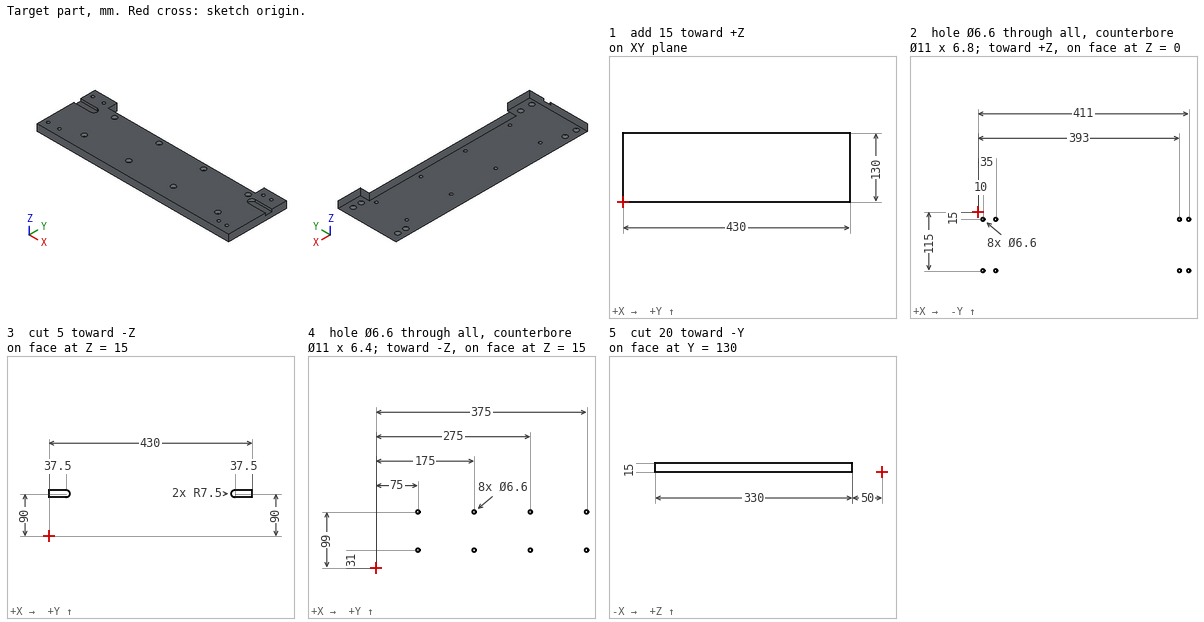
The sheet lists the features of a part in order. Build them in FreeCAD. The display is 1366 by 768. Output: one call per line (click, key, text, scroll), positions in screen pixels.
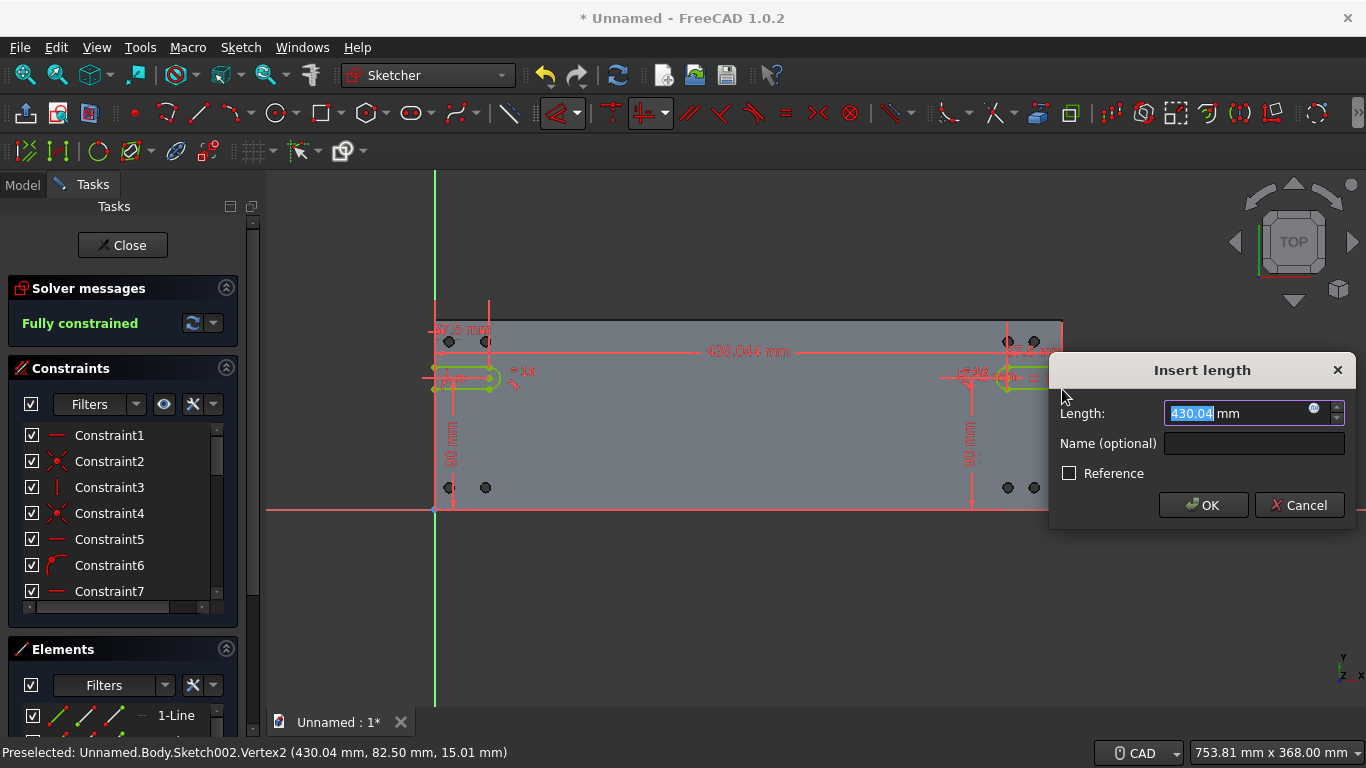
text(430)
key(Return)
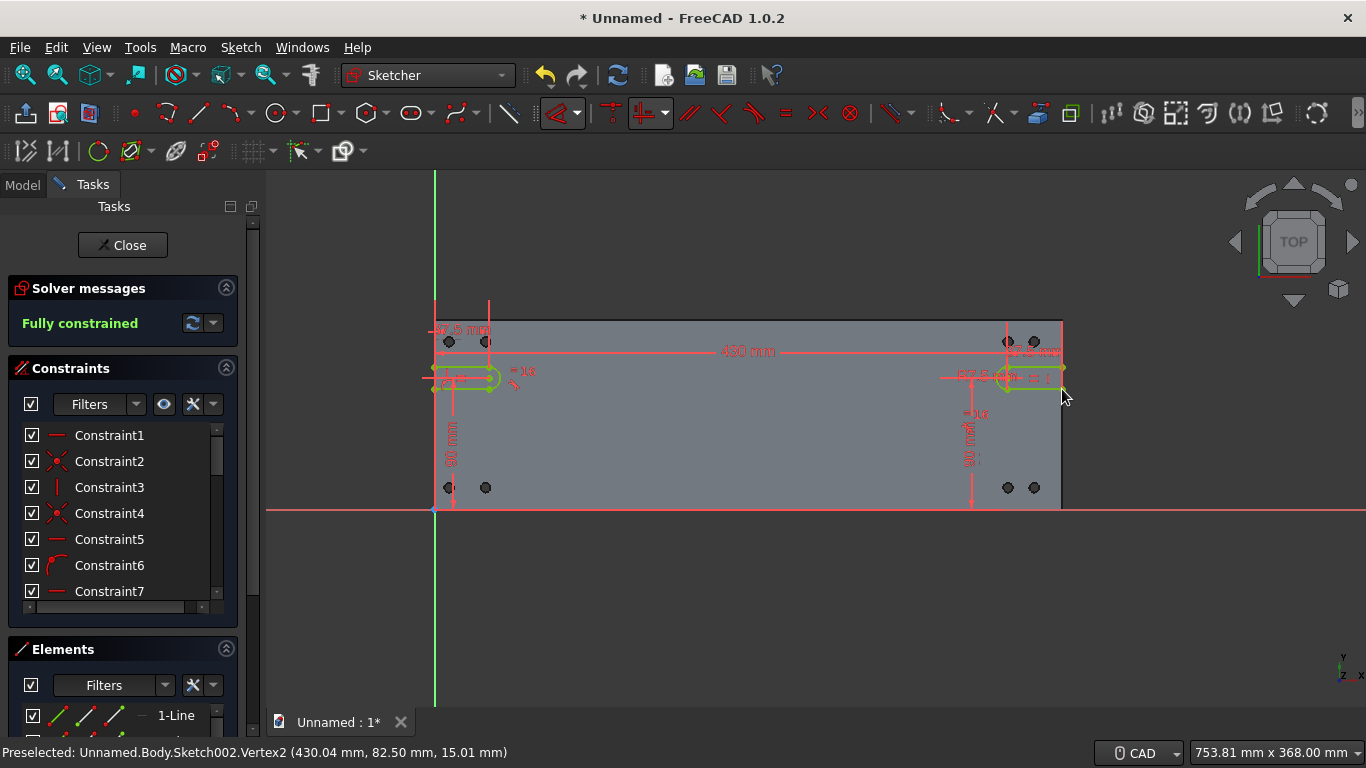
click(123, 245)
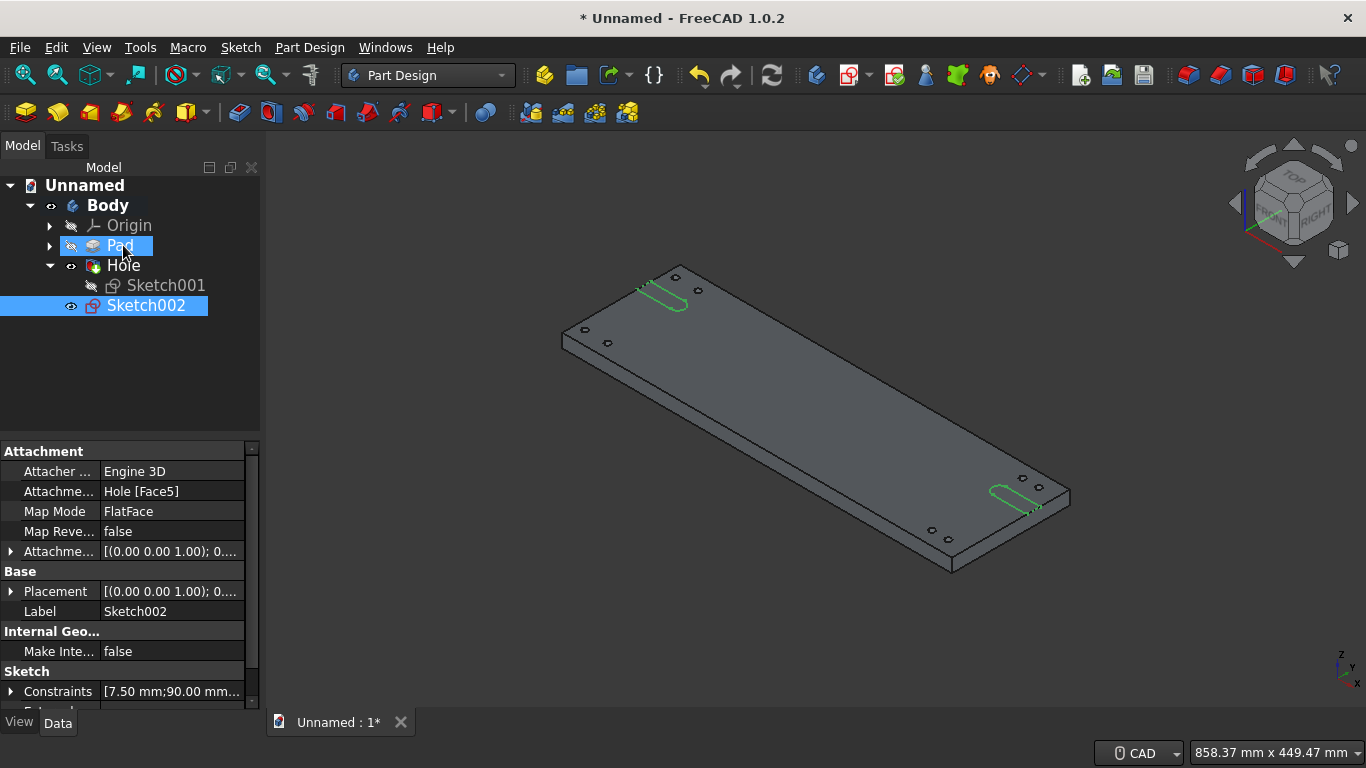
click(240, 112)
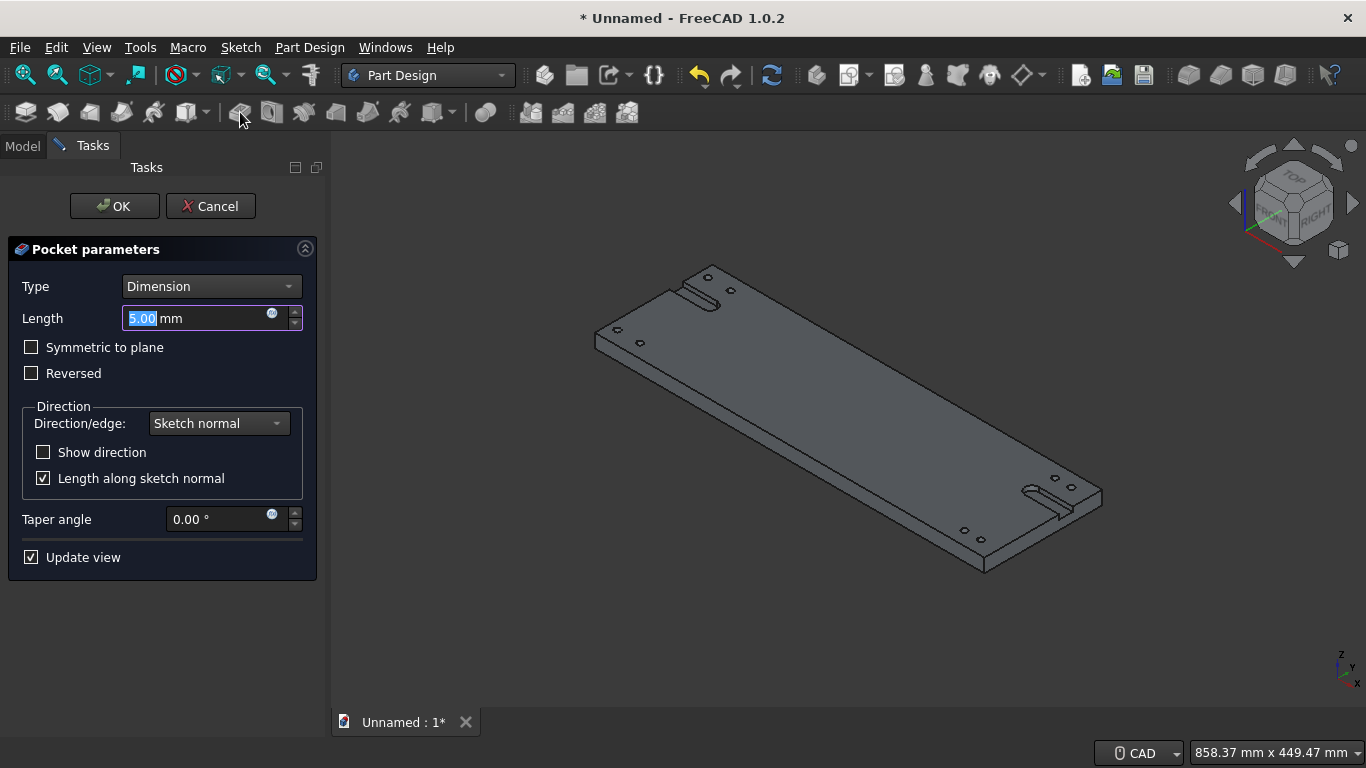
text(5)
key(Tab)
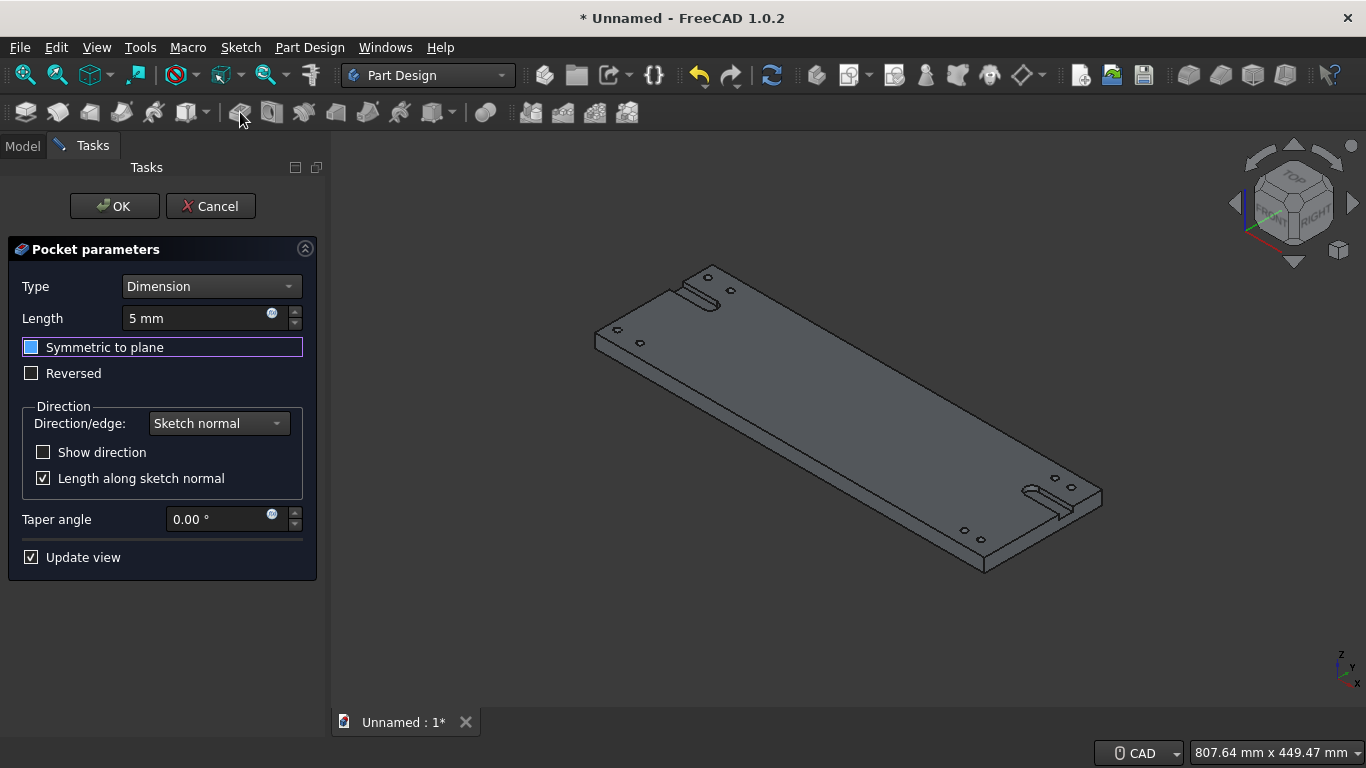
click(115, 206)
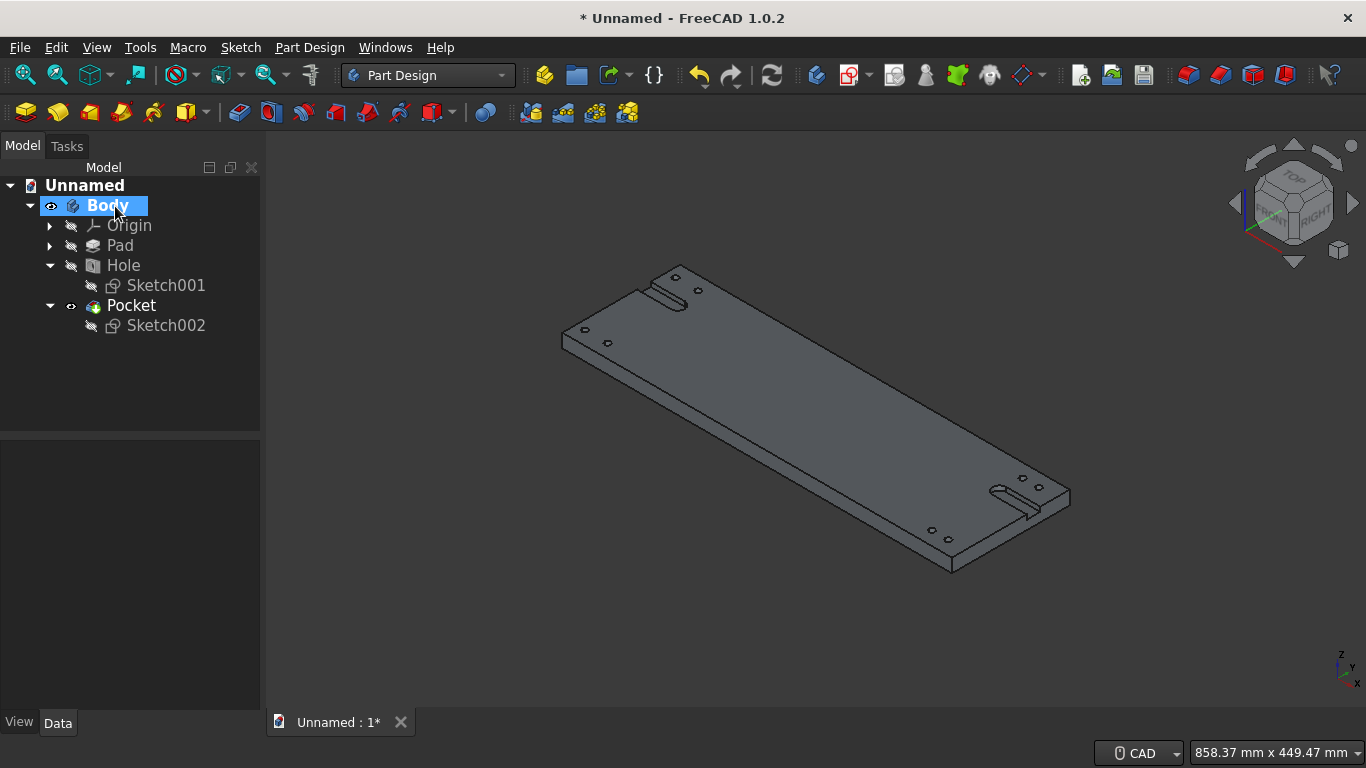
click(872, 442)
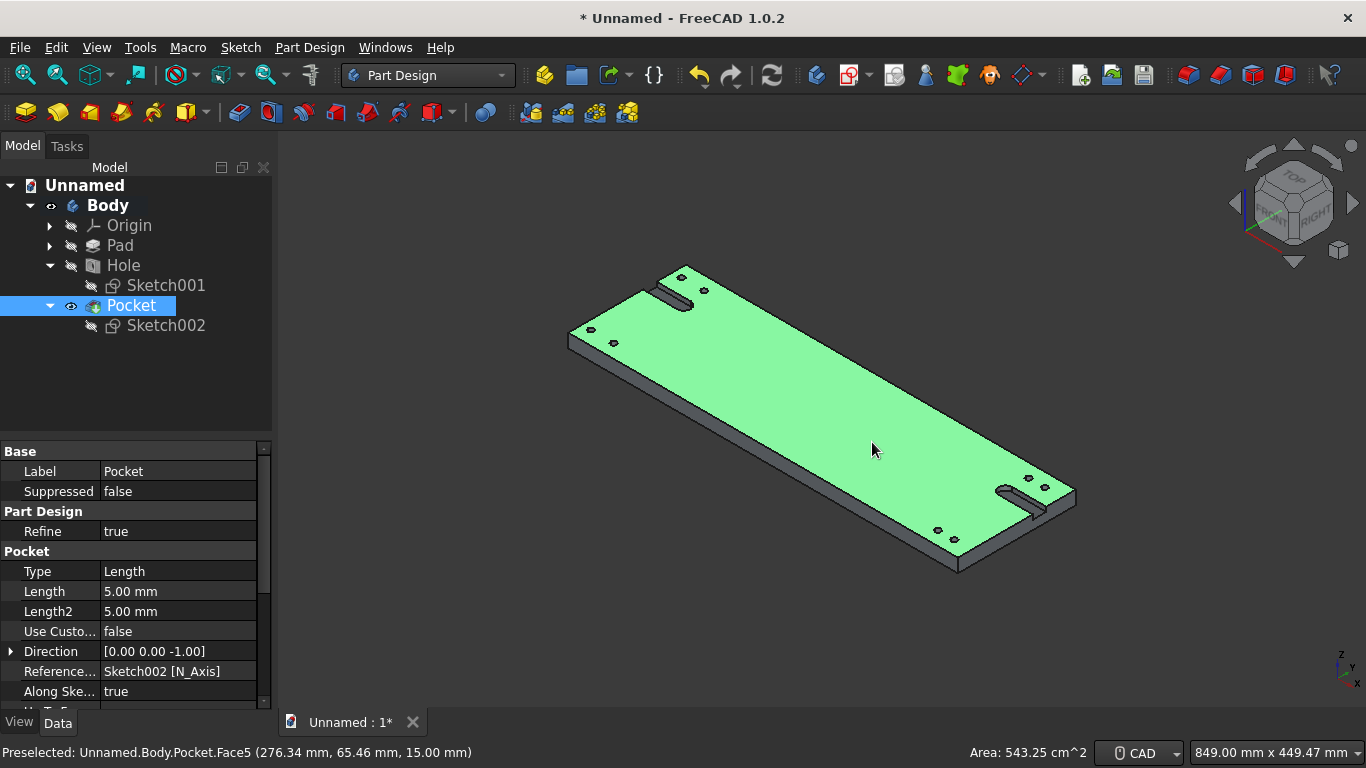
click(850, 76)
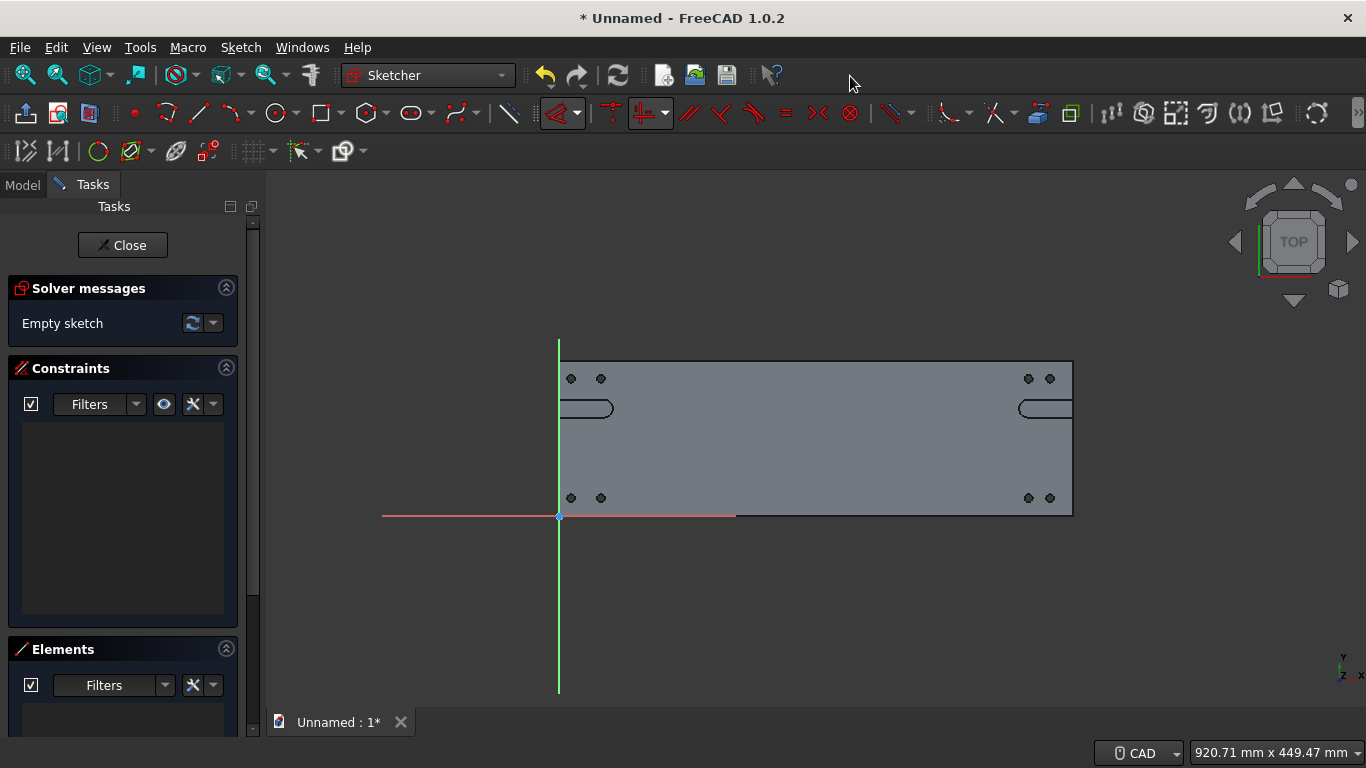
scroll(862, 489, up, 2)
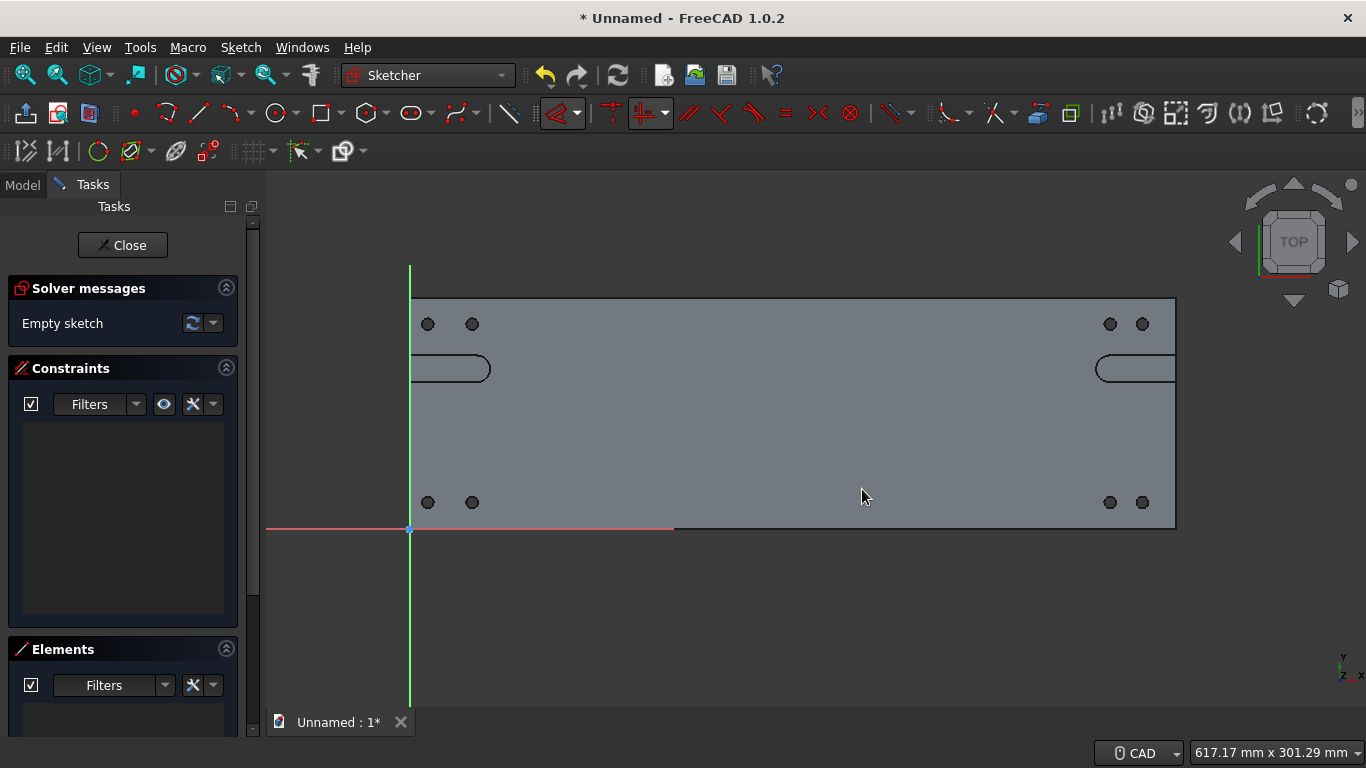
click(276, 114)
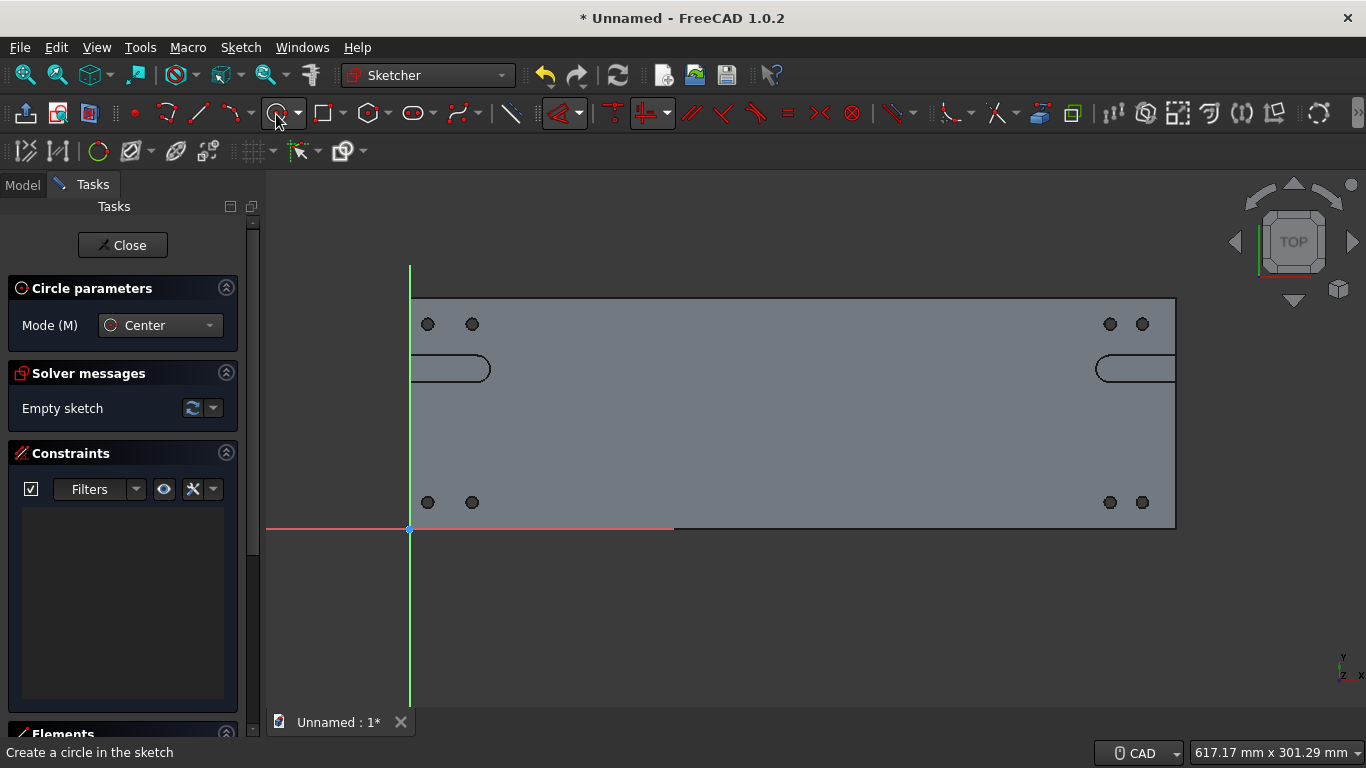
scroll(544, 353, up, 7)